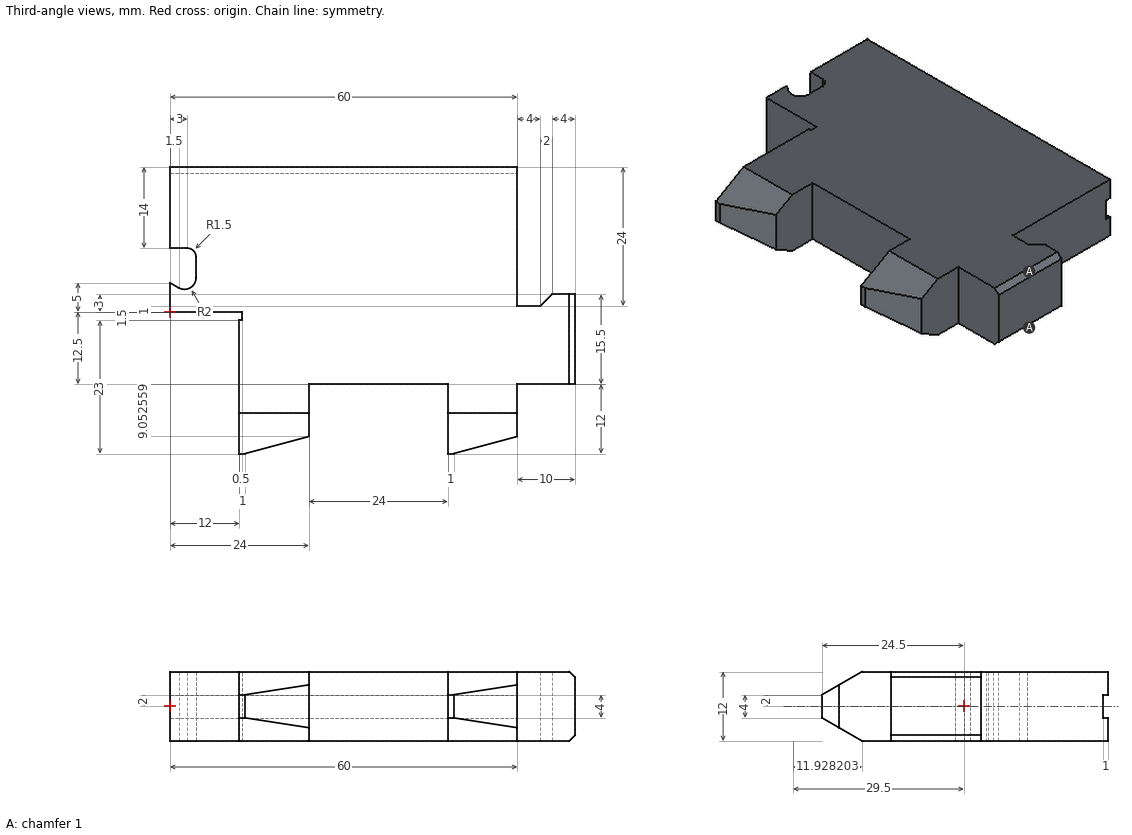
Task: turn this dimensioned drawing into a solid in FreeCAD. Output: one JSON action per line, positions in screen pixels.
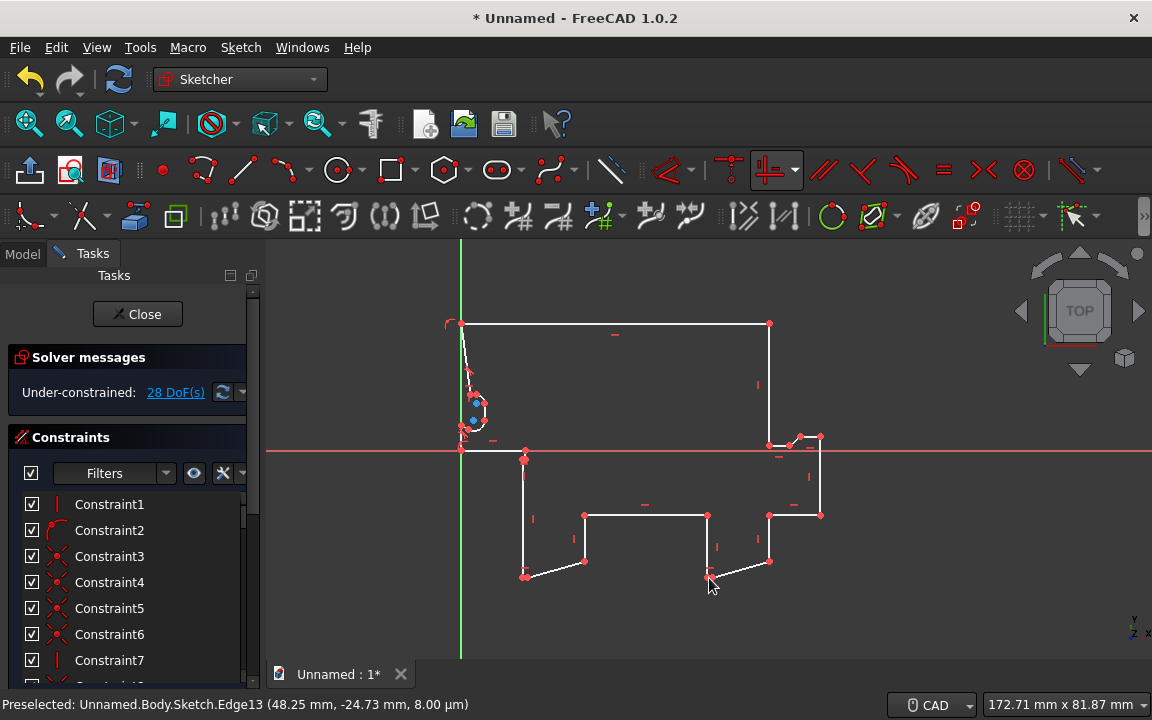
{"action": "scroll", "coordinate": [464, 345], "scroll_direction": "up", "scroll_amount": 8}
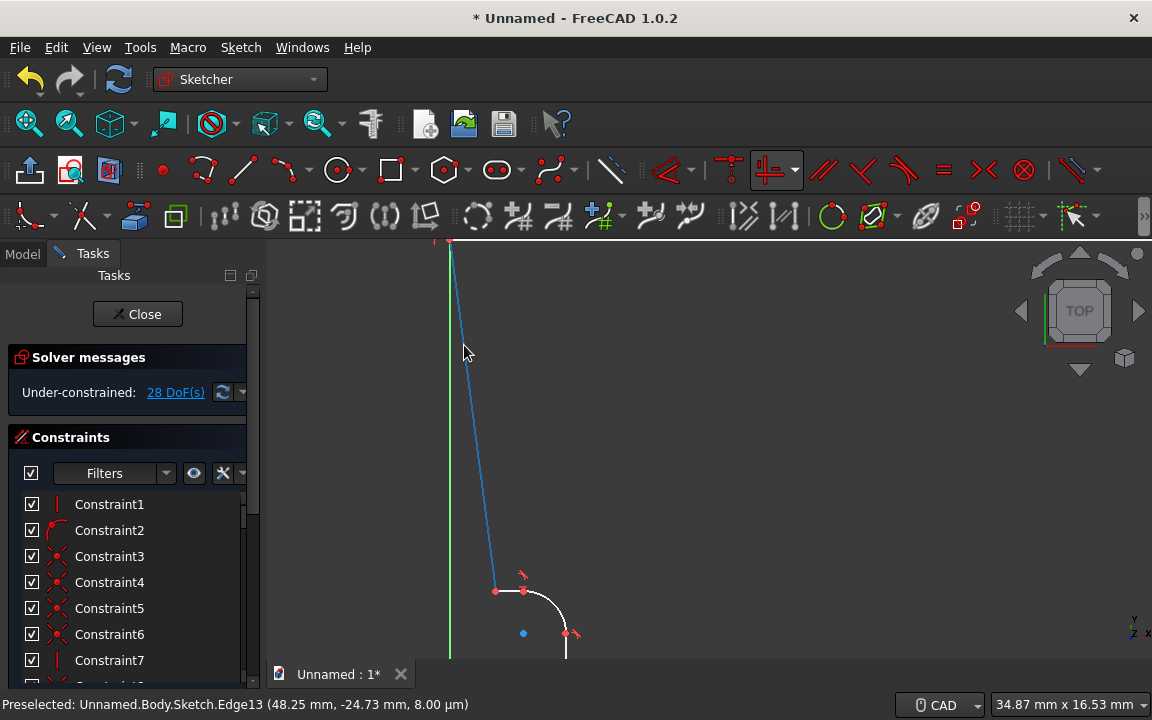
{"action": "left_click", "coordinate": [464, 345]}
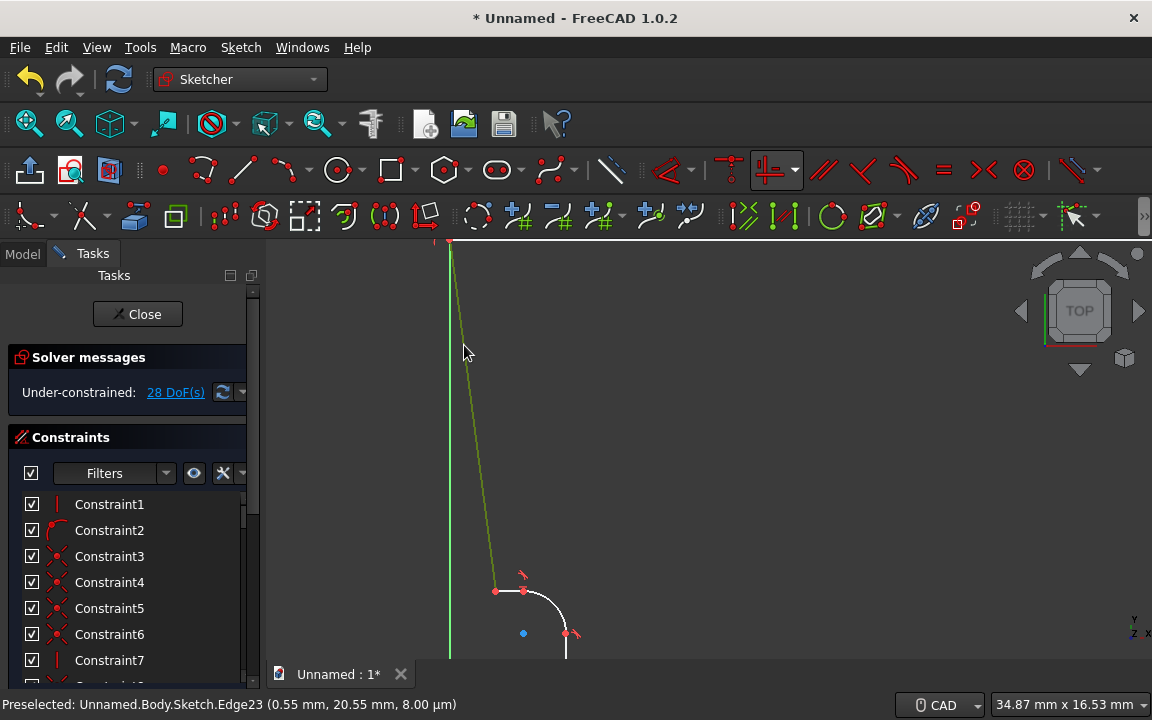
{"action": "left_click", "coordinate": [798, 170]}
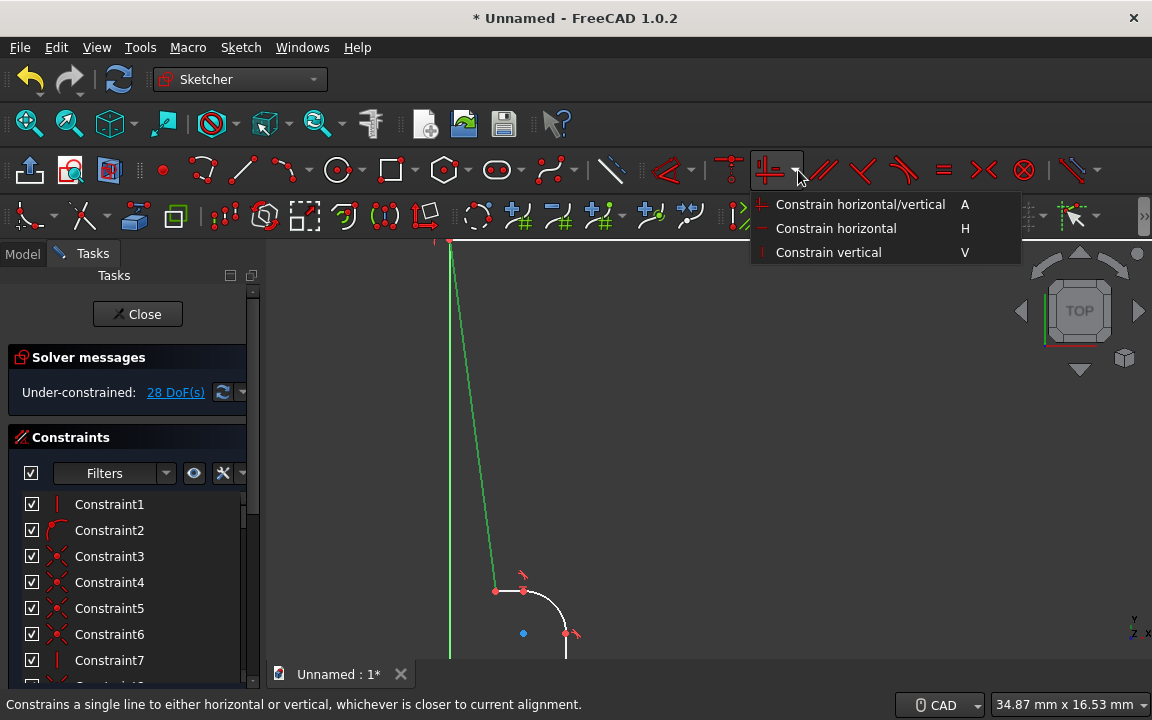
{"action": "left_click", "coordinate": [886, 252]}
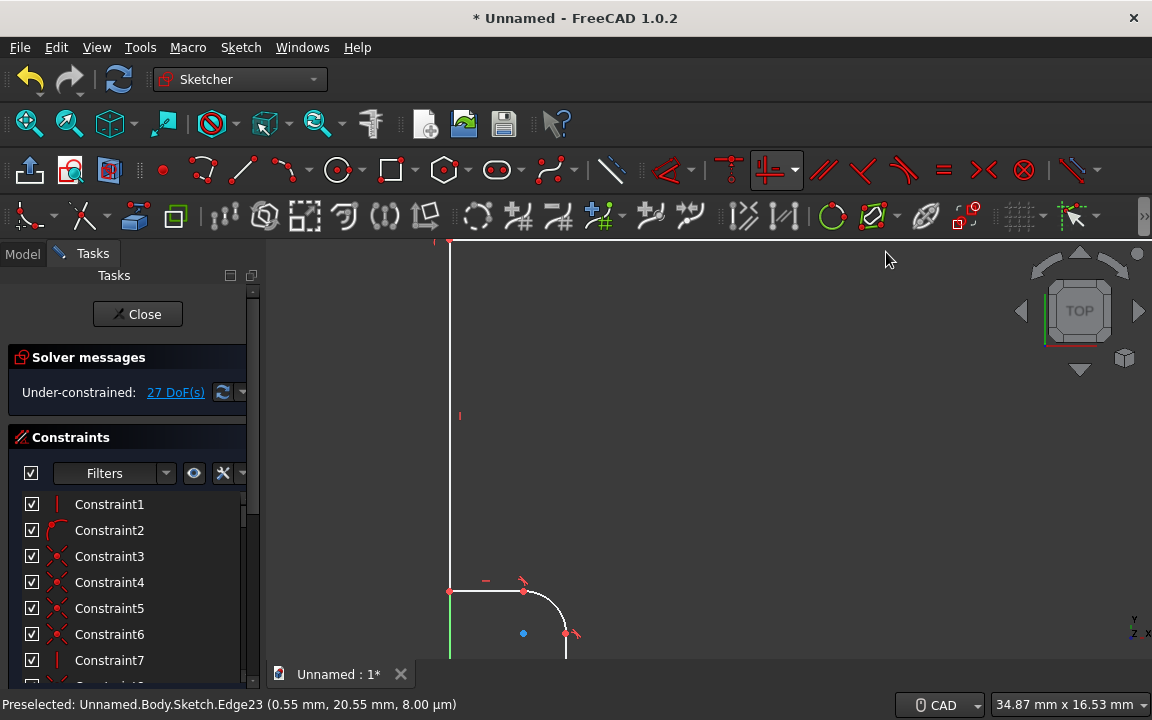
{"action": "left_click", "coordinate": [666, 170]}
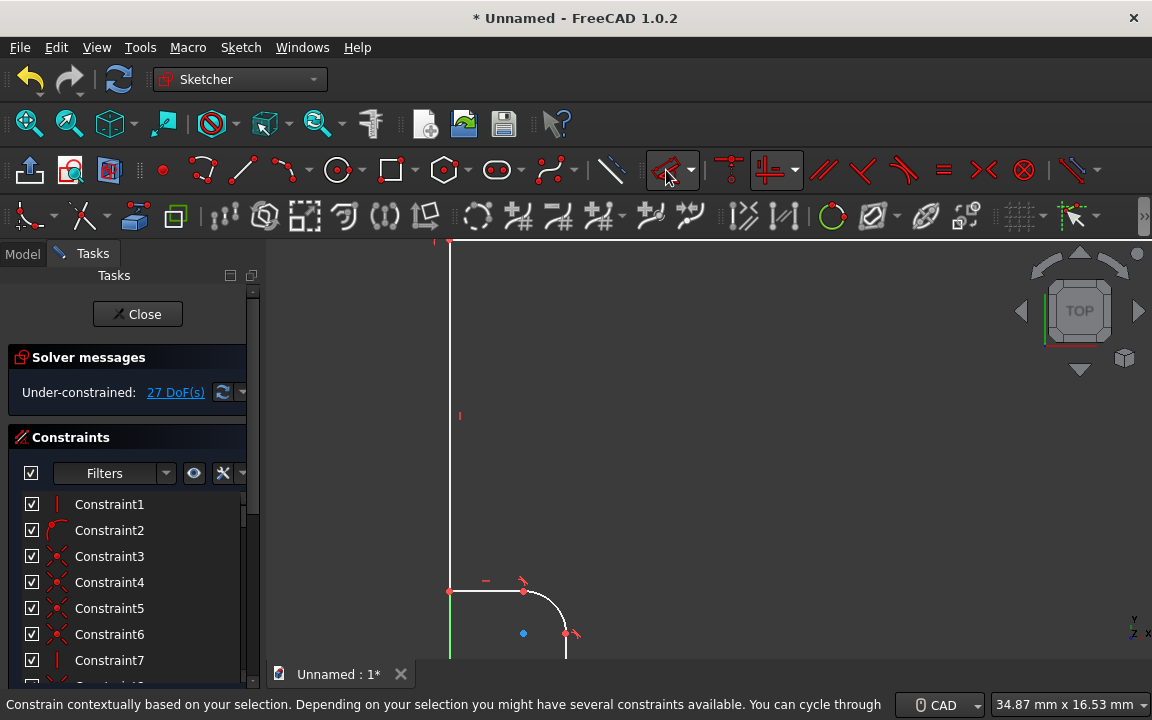
{"action": "scroll", "coordinate": [464, 345], "scroll_direction": "down", "scroll_amount": 8}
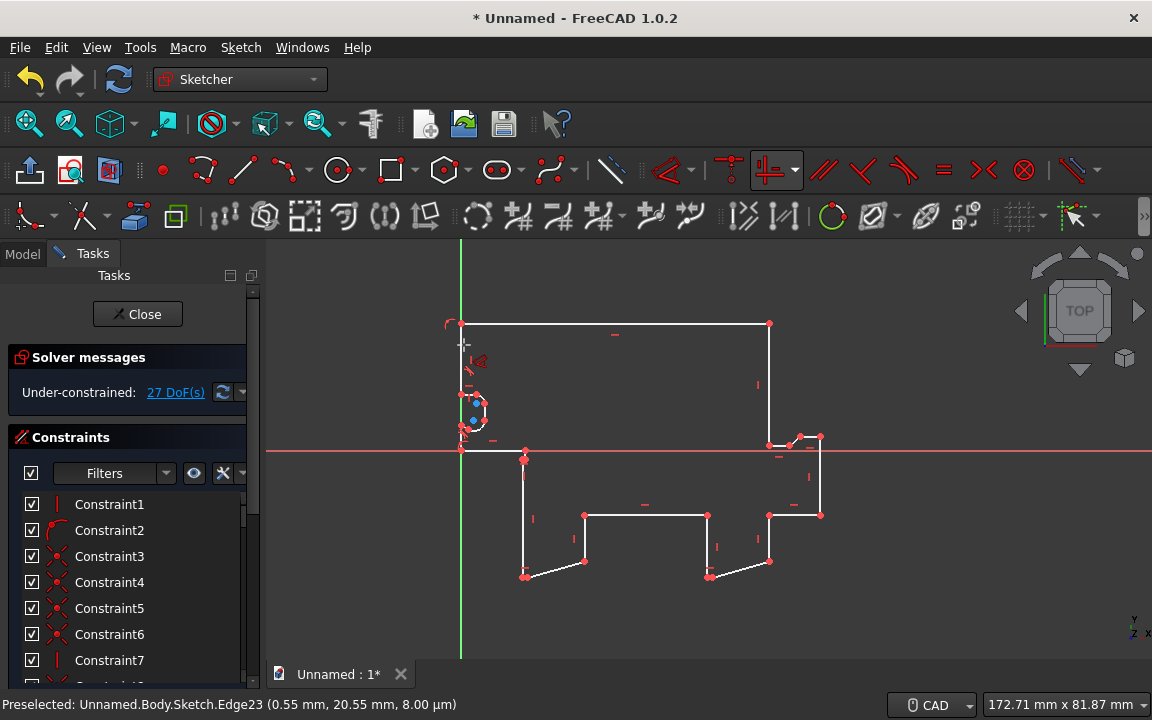
{"action": "scroll", "coordinate": [475, 431], "scroll_direction": "up", "scroll_amount": 7}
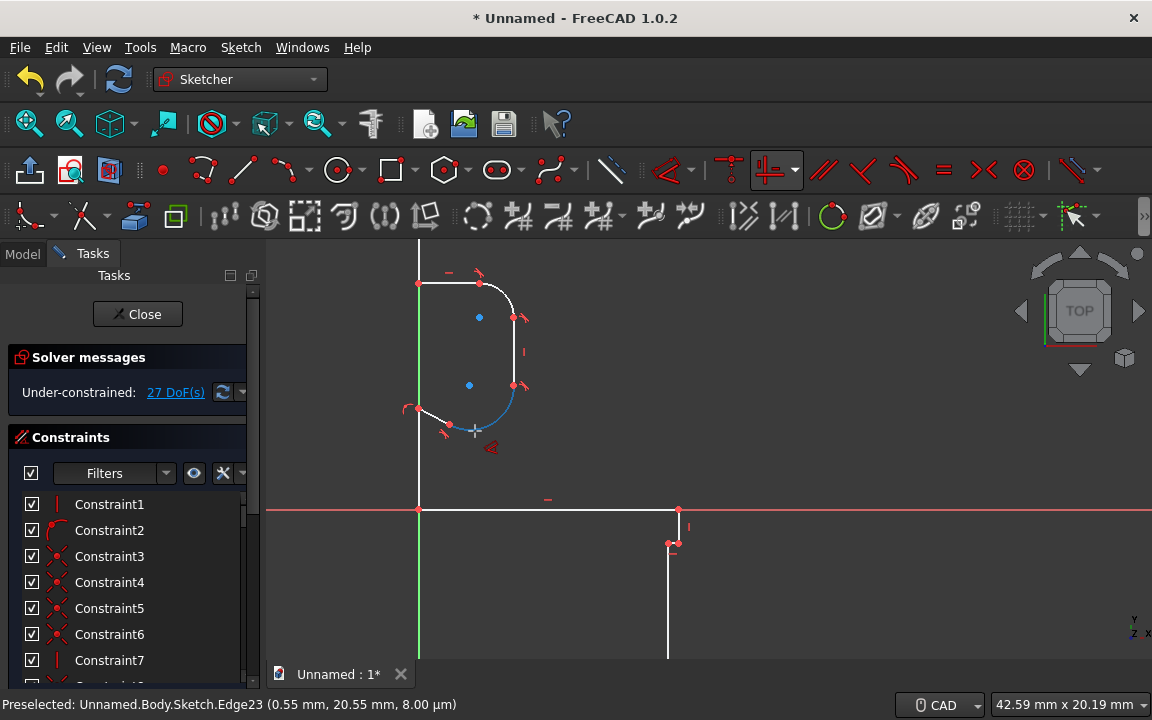
{"action": "left_click", "coordinate": [476, 429]}
{"action": "left_click", "coordinate": [480, 461]}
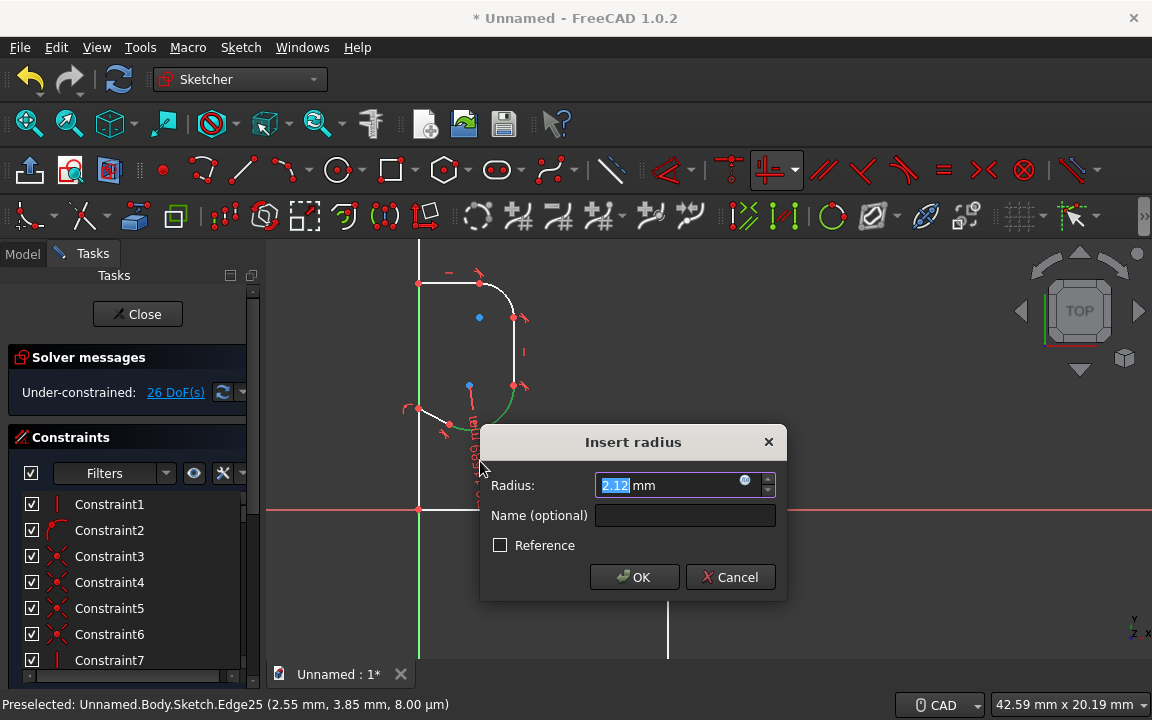
{"action": "type", "text": "2"}
{"action": "key", "text": "Return"}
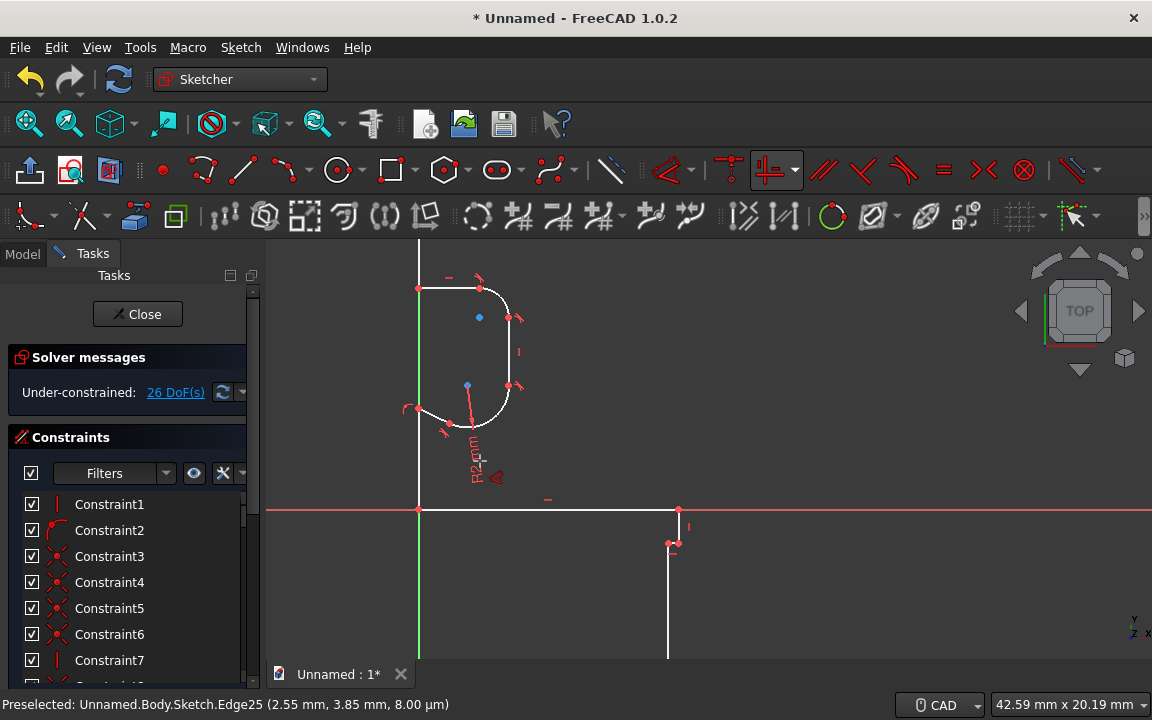
{"action": "scroll", "coordinate": [506, 304], "scroll_direction": "up", "scroll_amount": 2}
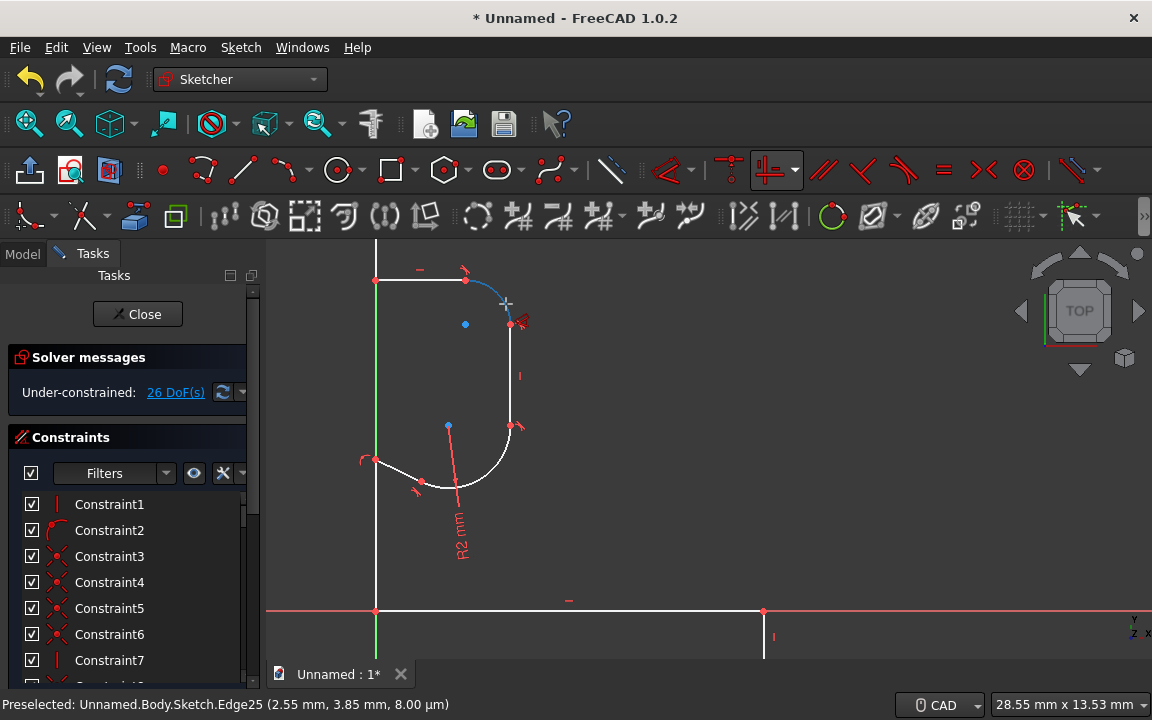
{"action": "left_click", "coordinate": [505, 305]}
{"action": "left_click", "coordinate": [534, 291]}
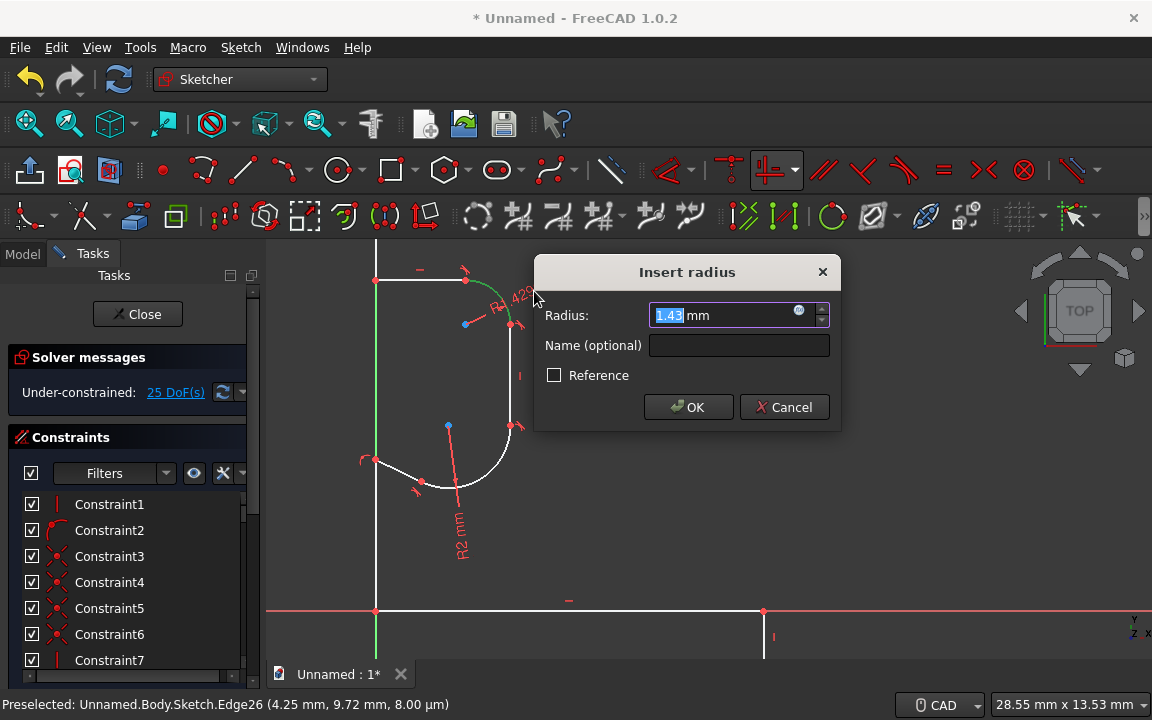
{"action": "type", "text": "1.5"}
{"action": "key", "text": "Return"}